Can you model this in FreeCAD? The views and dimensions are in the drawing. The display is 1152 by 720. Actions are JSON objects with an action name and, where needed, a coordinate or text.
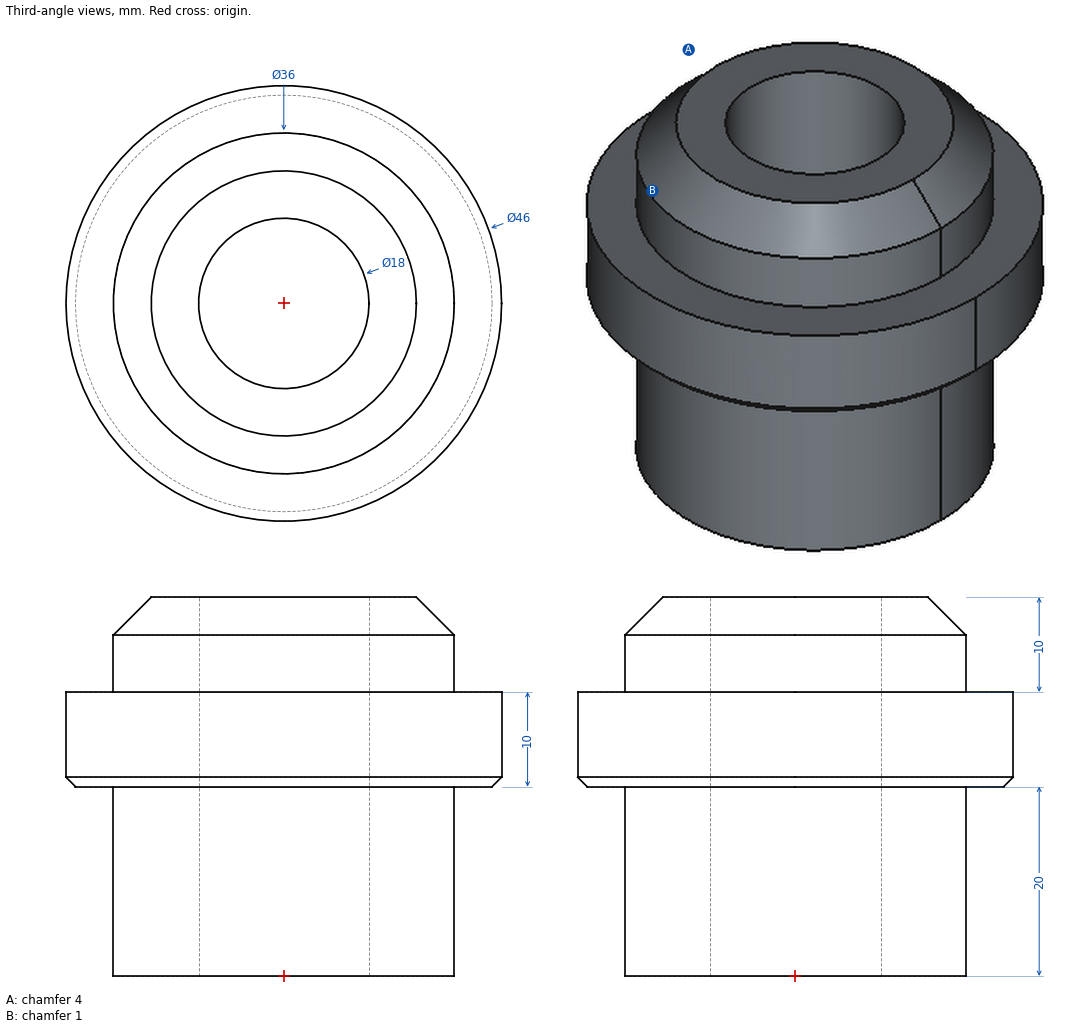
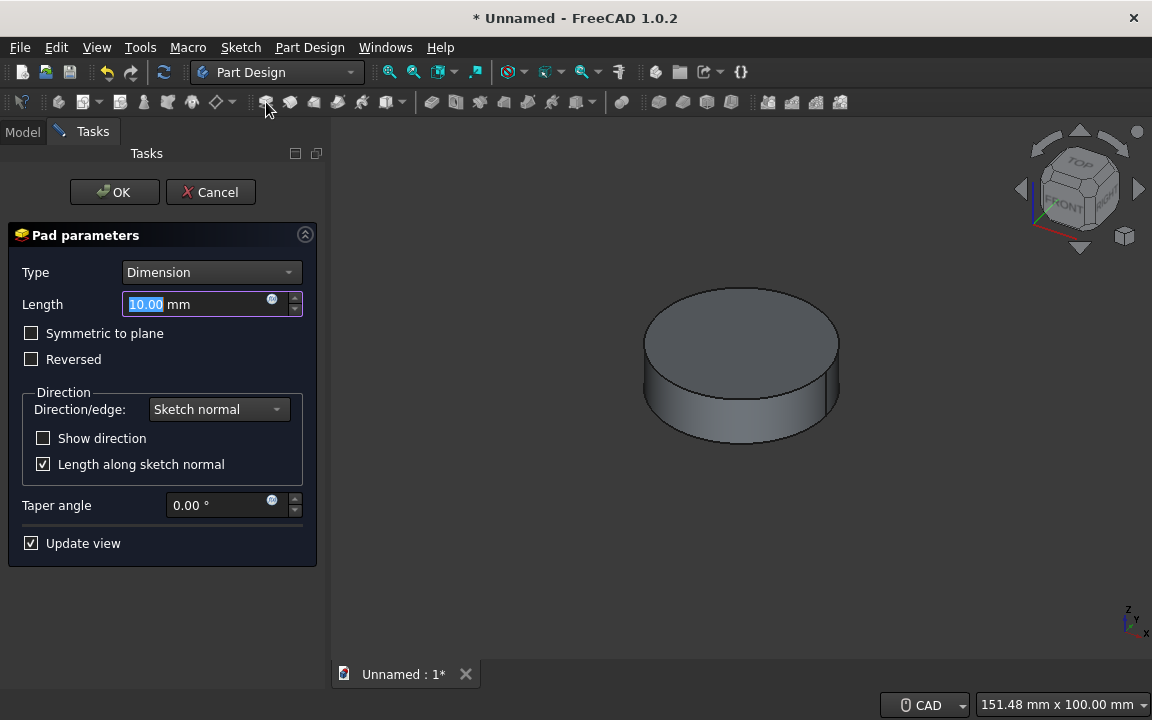
{"action": "type", "text": "20"}
{"action": "key", "text": "Tab"}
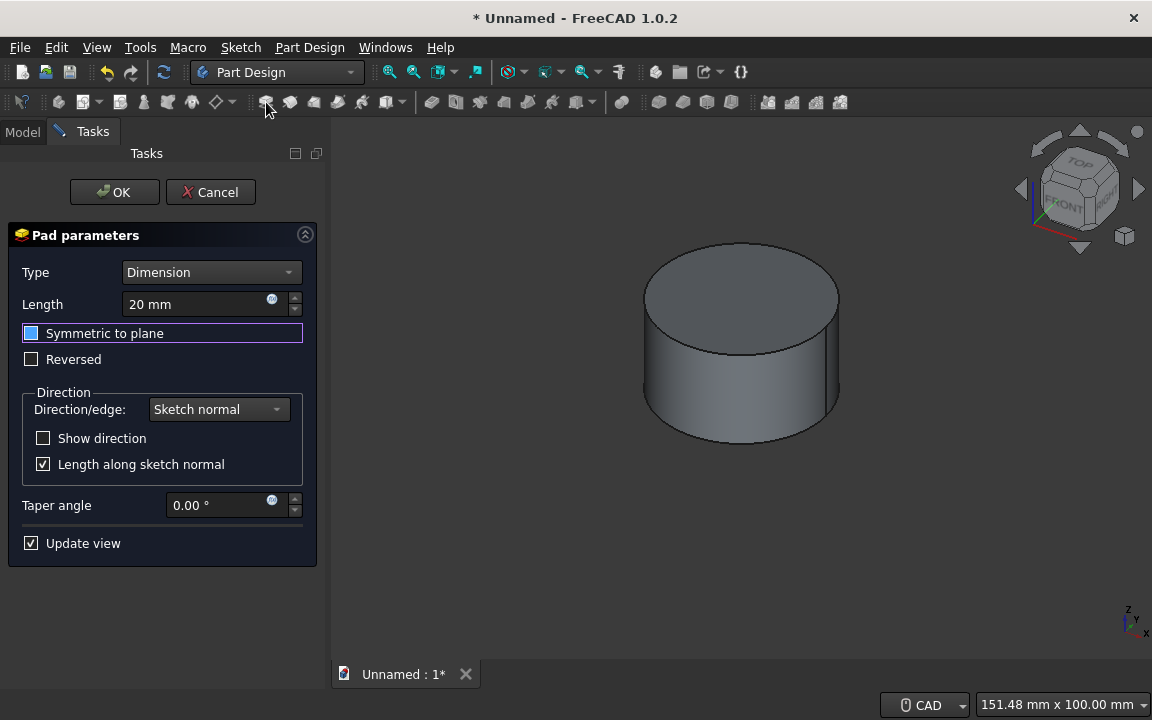
{"action": "left_click", "coordinate": [115, 192]}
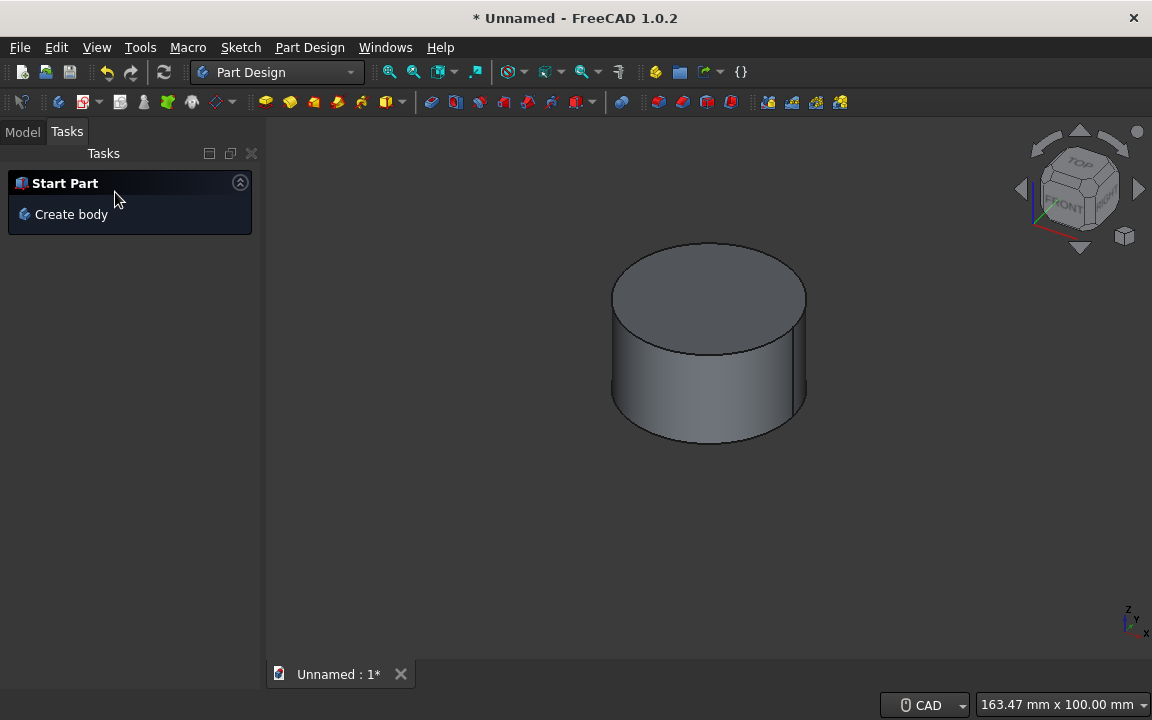
{"action": "key", "text": "v f"}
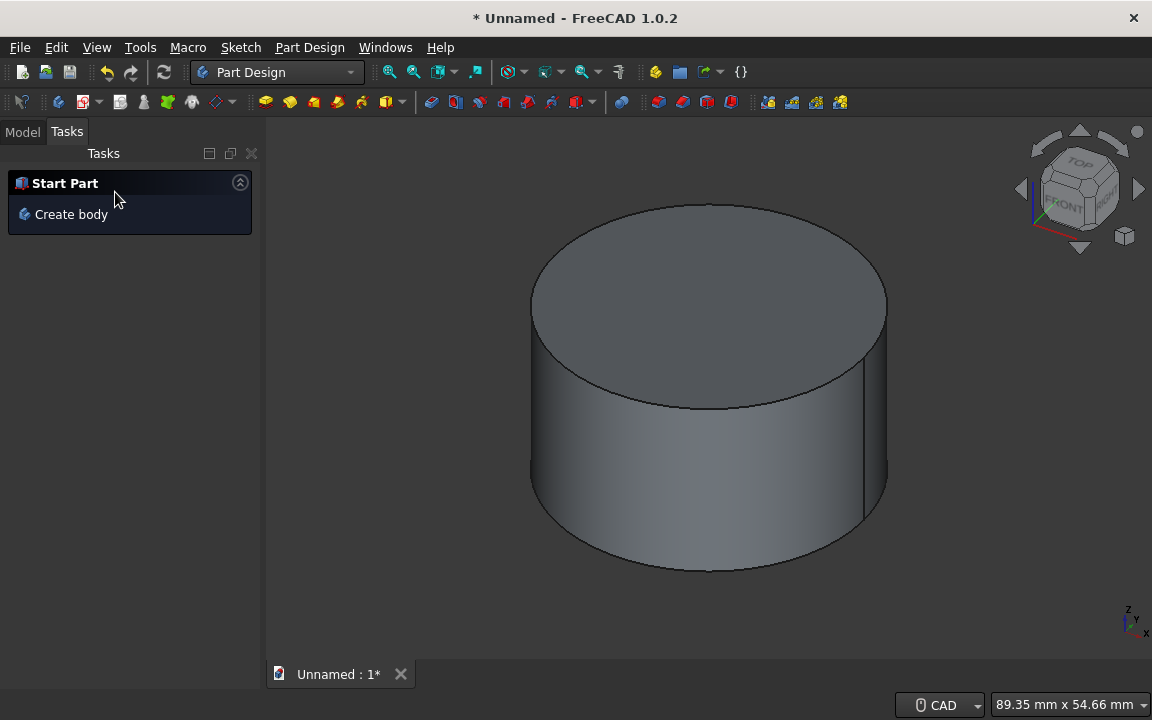
{"action": "left_click", "coordinate": [709, 306]}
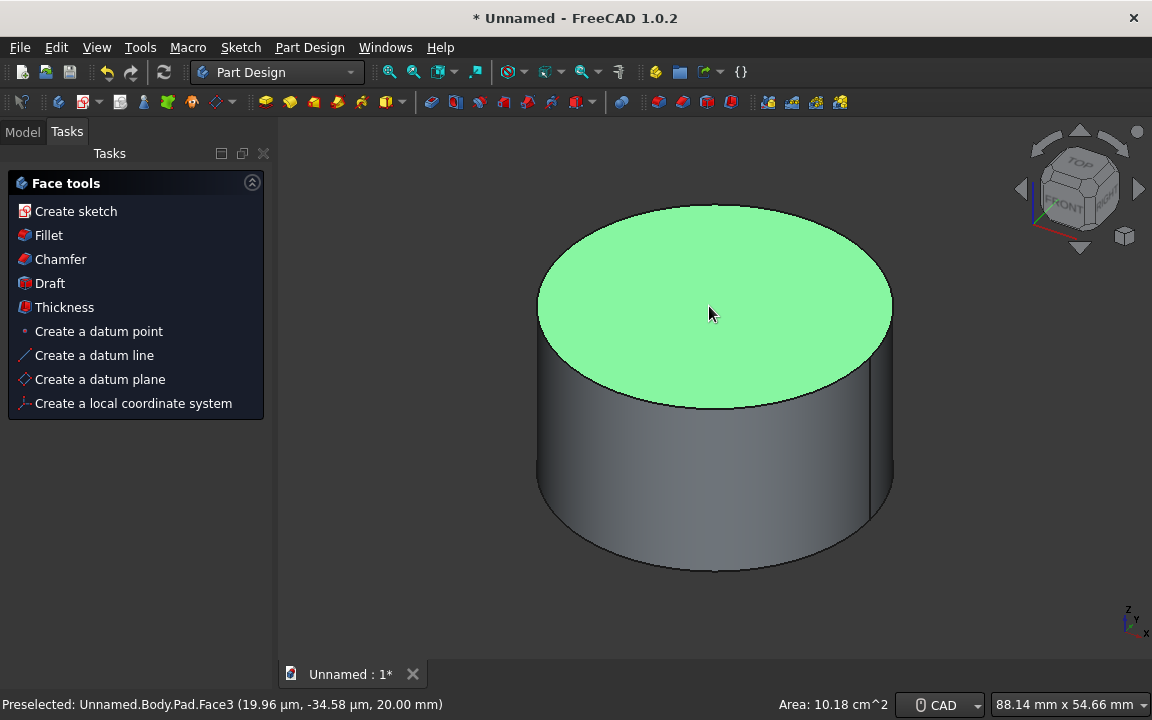
{"action": "left_click", "coordinate": [84, 102]}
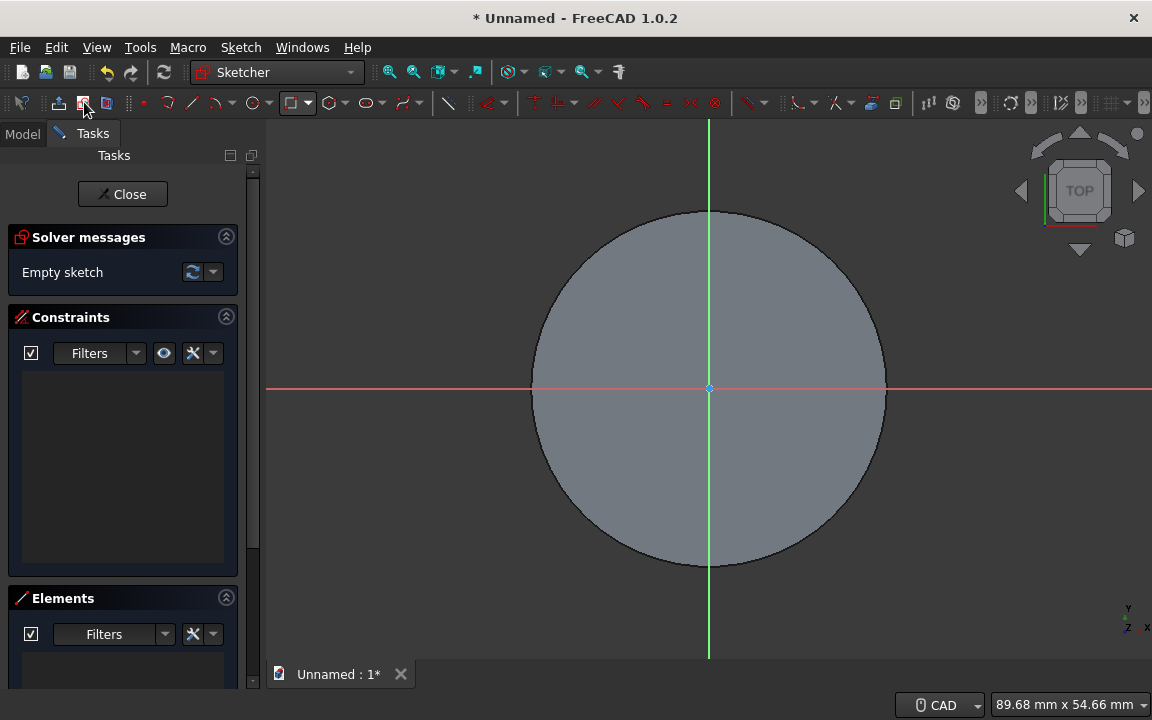
{"action": "scroll", "coordinate": [331, 389], "scroll_direction": "down", "scroll_amount": 1}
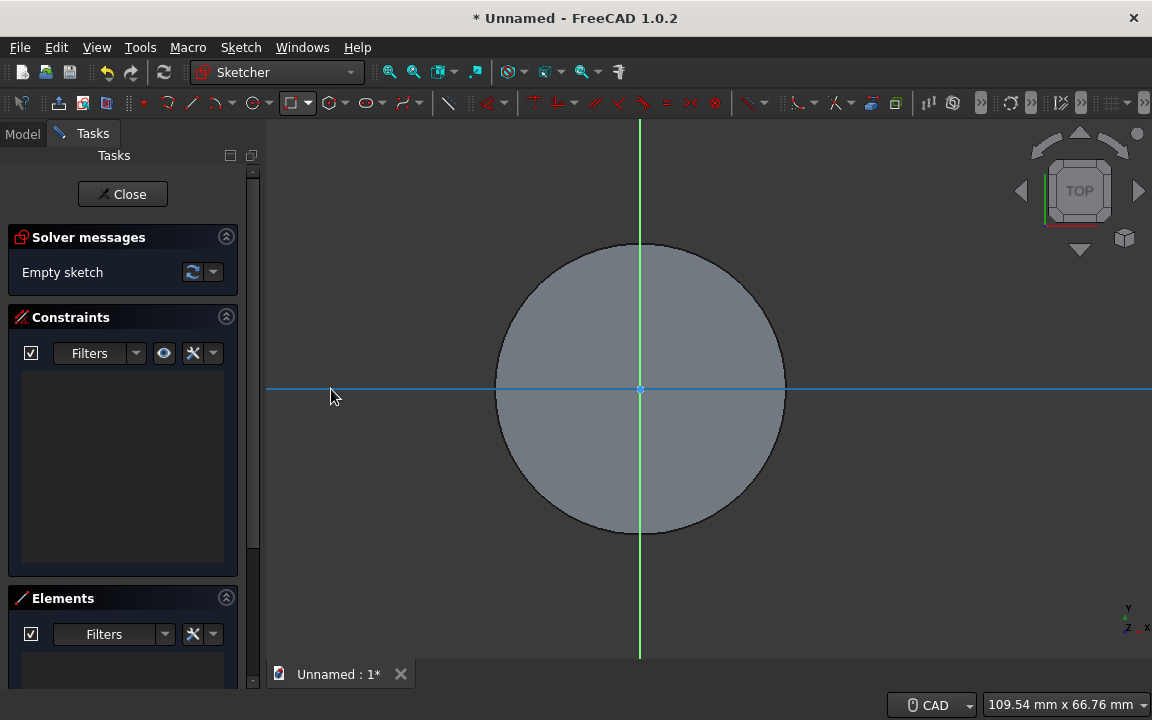
{"action": "key", "text": "g c"}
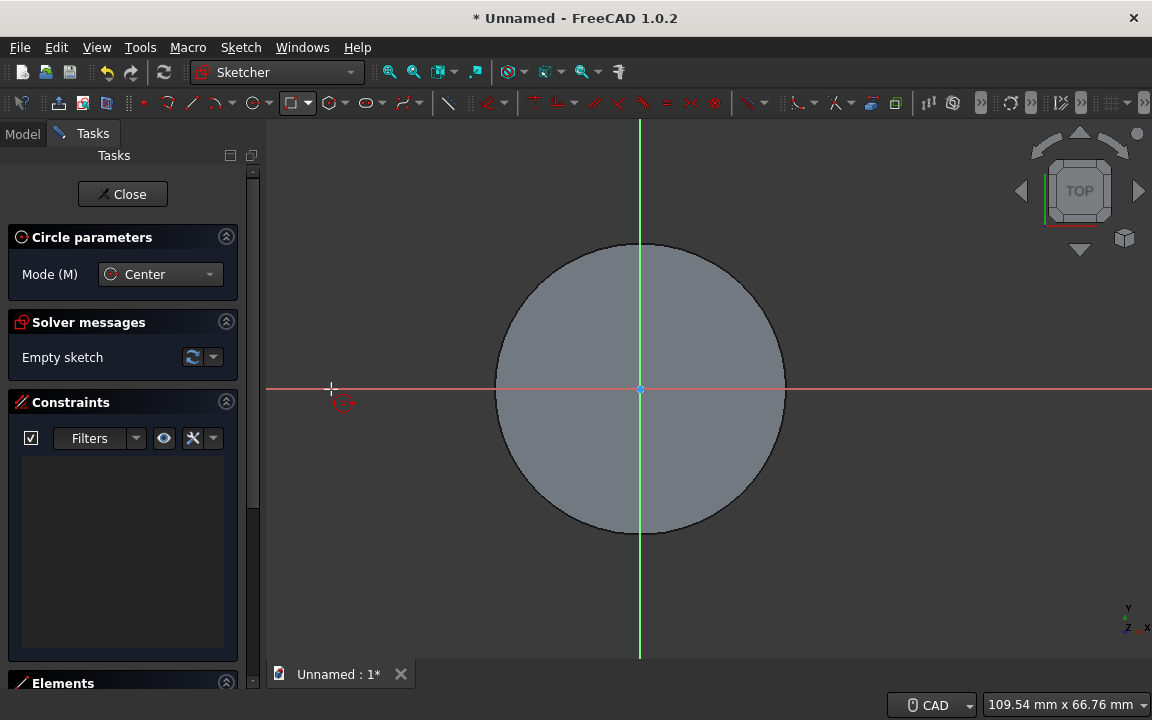
{"action": "left_click", "coordinate": [640, 389]}
{"action": "left_click", "coordinate": [772, 258]}
{"action": "key", "text": "Escape"}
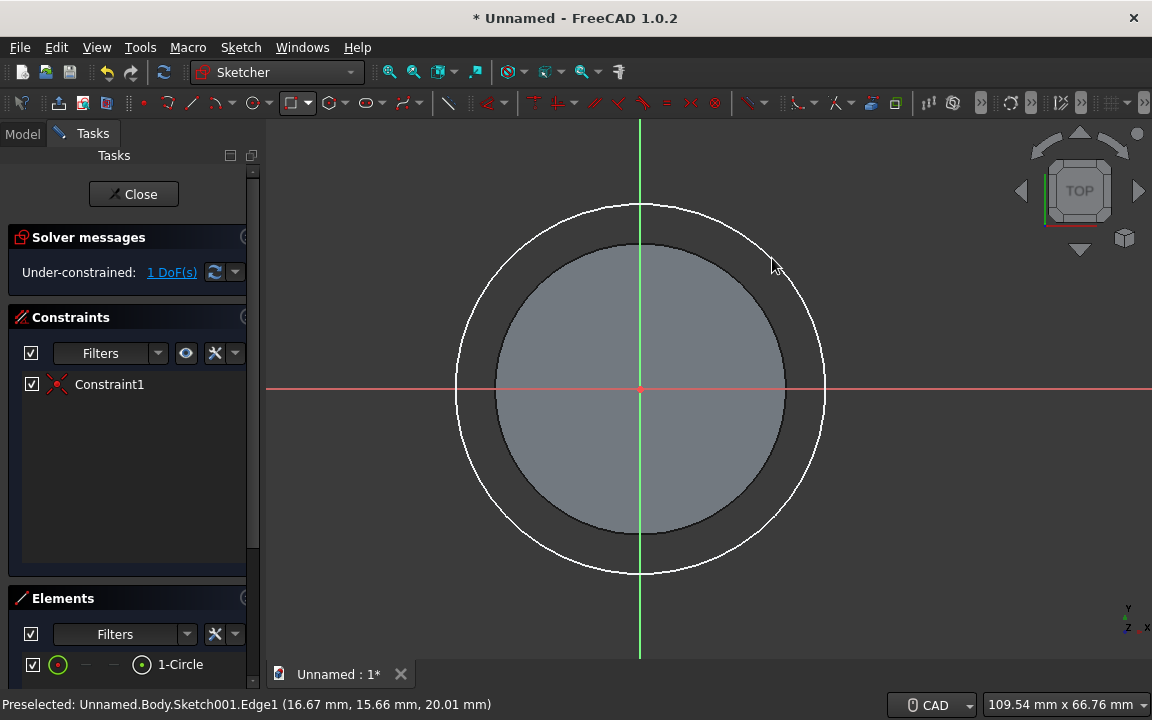
{"action": "left_click", "coordinate": [488, 104]}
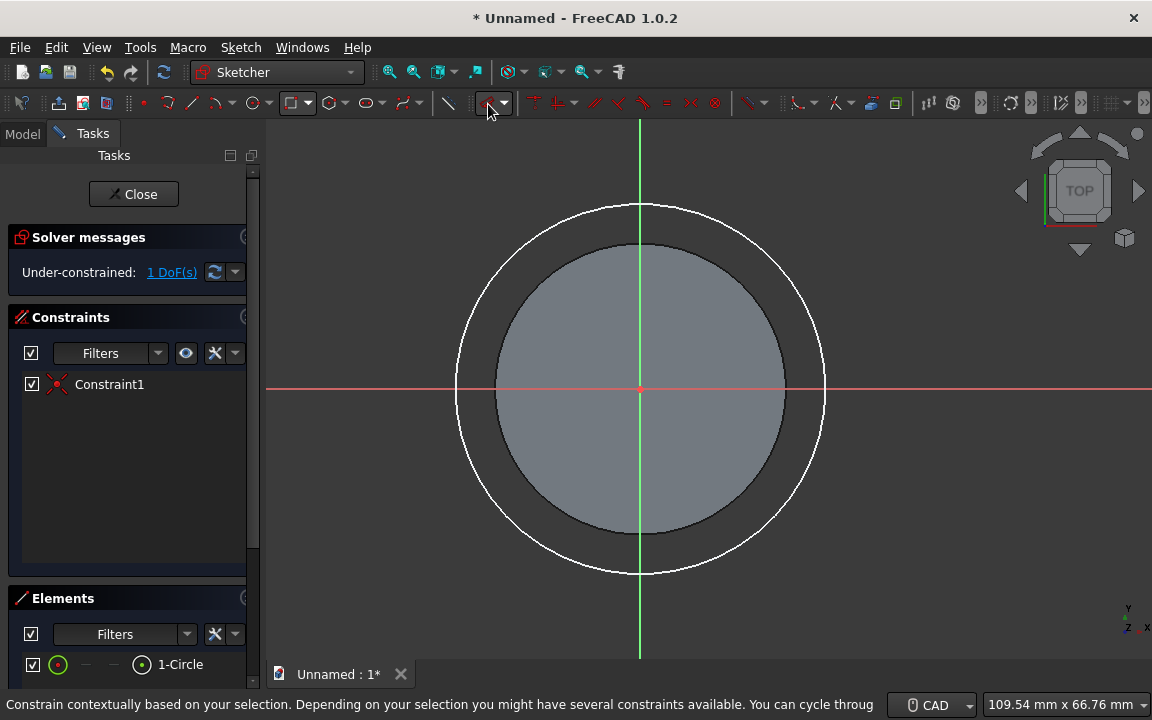
{"action": "left_click", "coordinate": [771, 258]}
{"action": "left_click", "coordinate": [794, 235]}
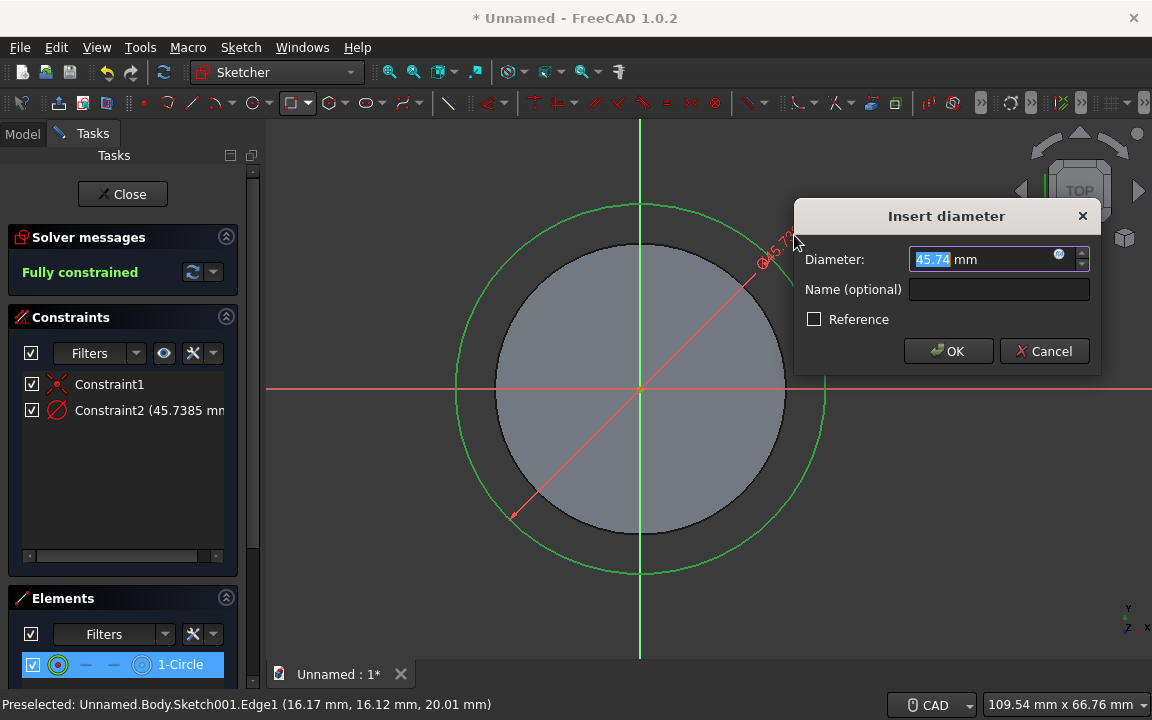
{"action": "type", "text": "46"}
{"action": "key", "text": "Return"}
{"action": "key", "text": "Escape"}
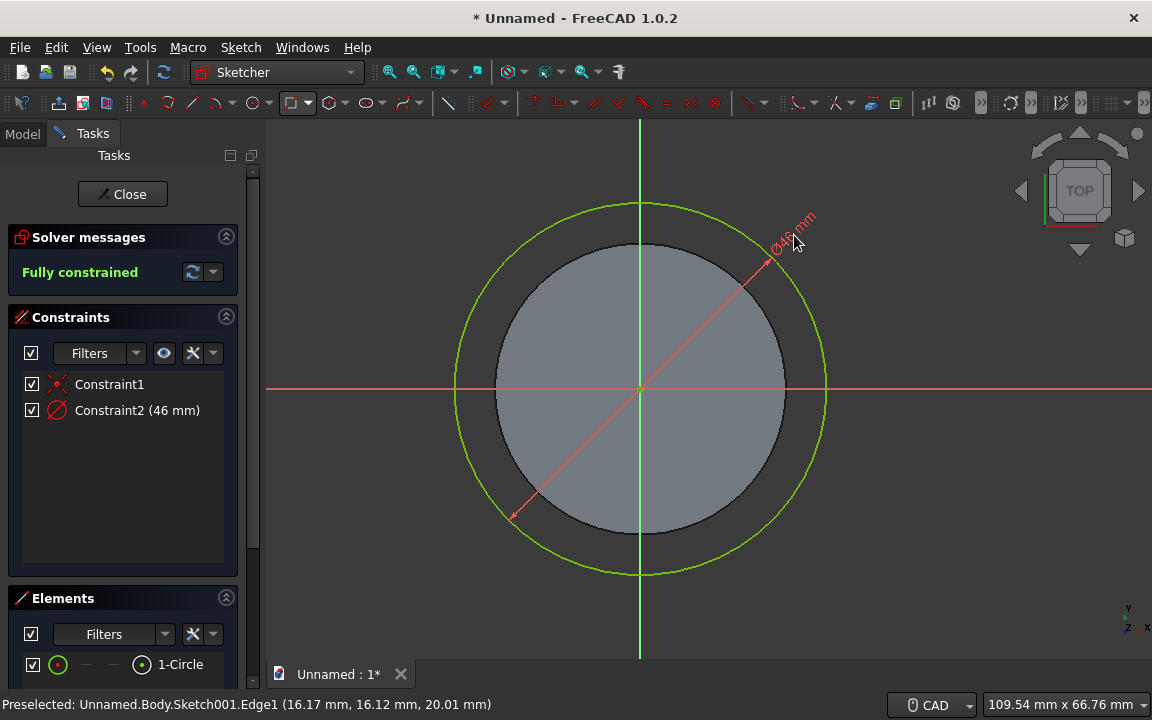
{"action": "left_click", "coordinate": [123, 194]}